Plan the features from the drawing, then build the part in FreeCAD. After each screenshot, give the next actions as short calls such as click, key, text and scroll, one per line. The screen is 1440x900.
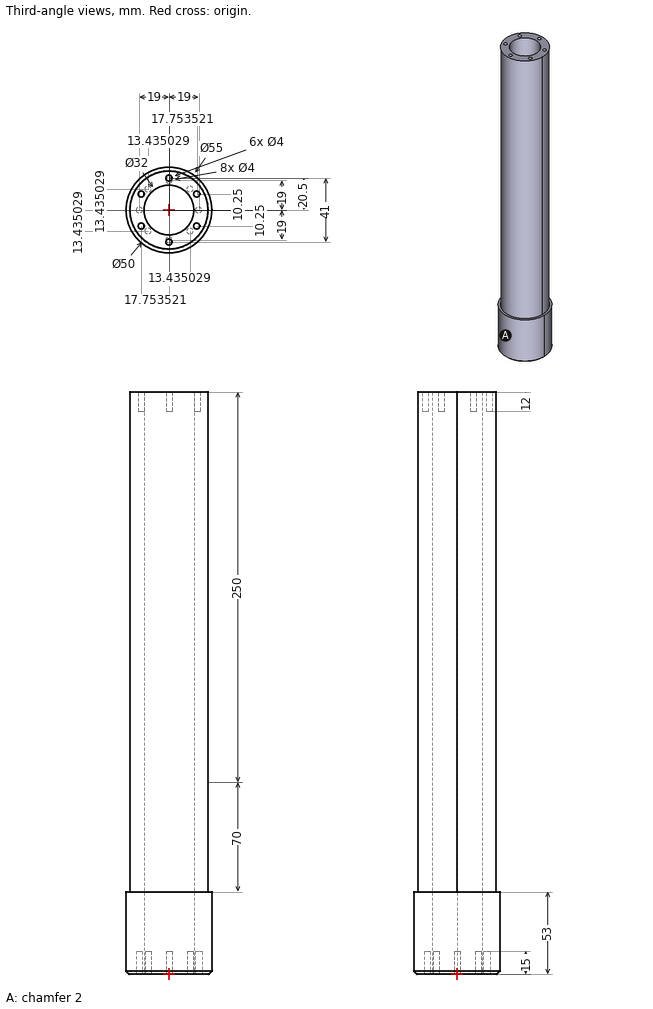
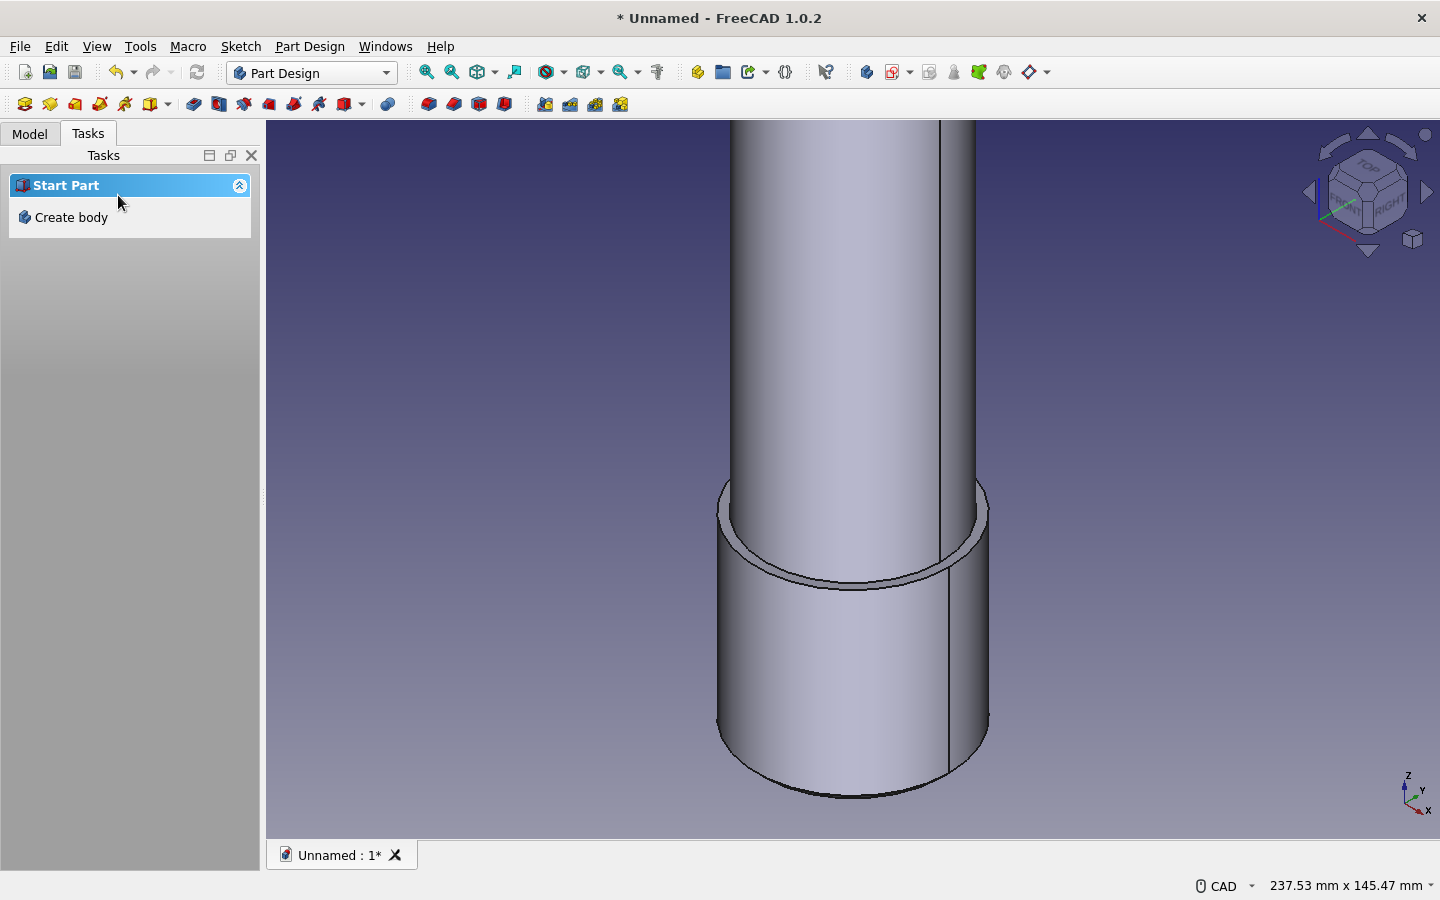
click(427, 72)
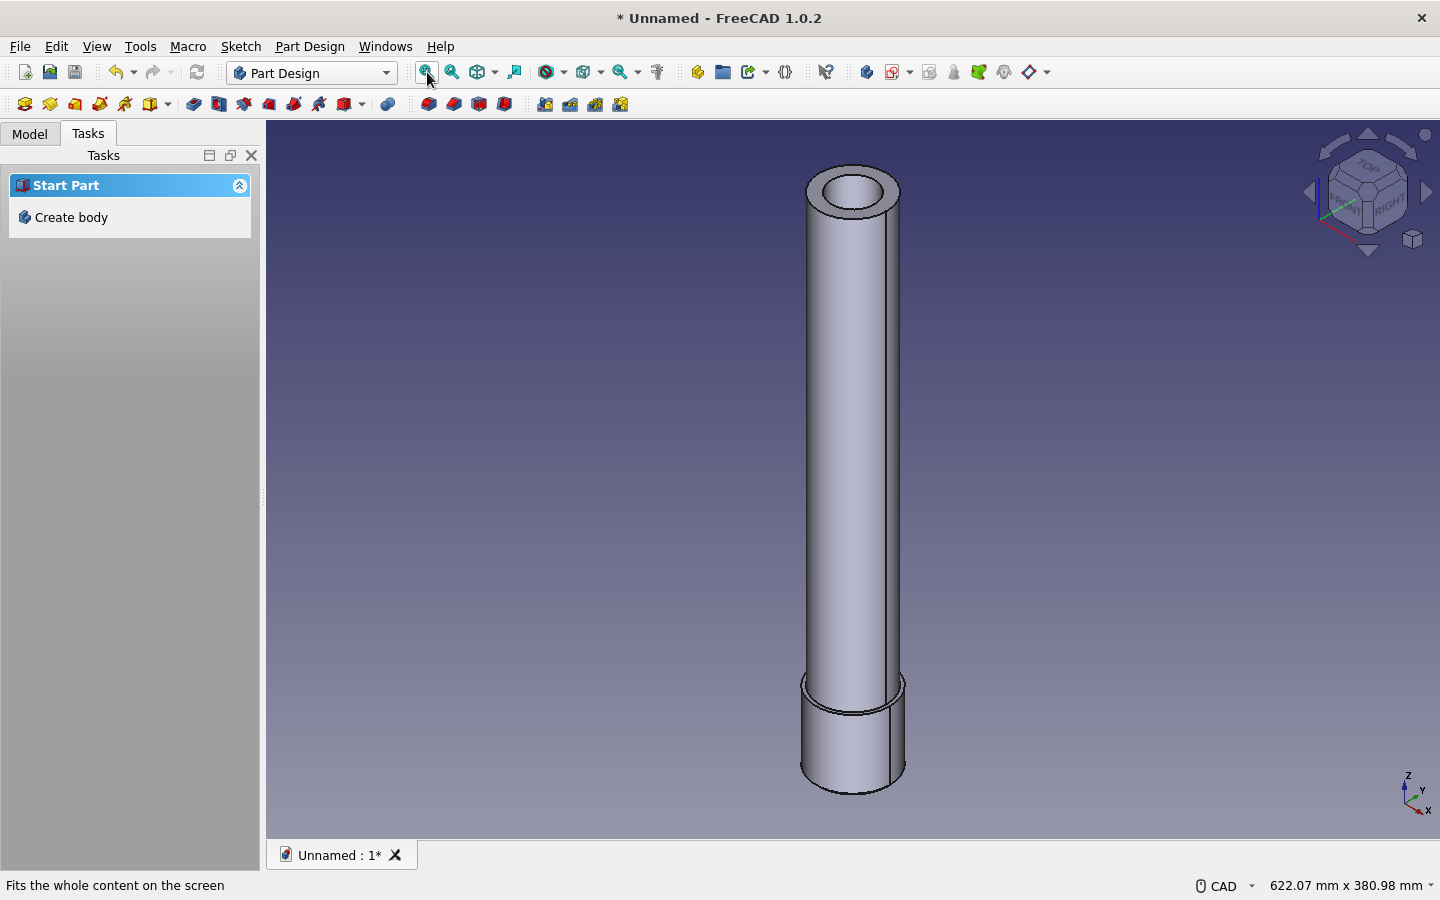
click(815, 191)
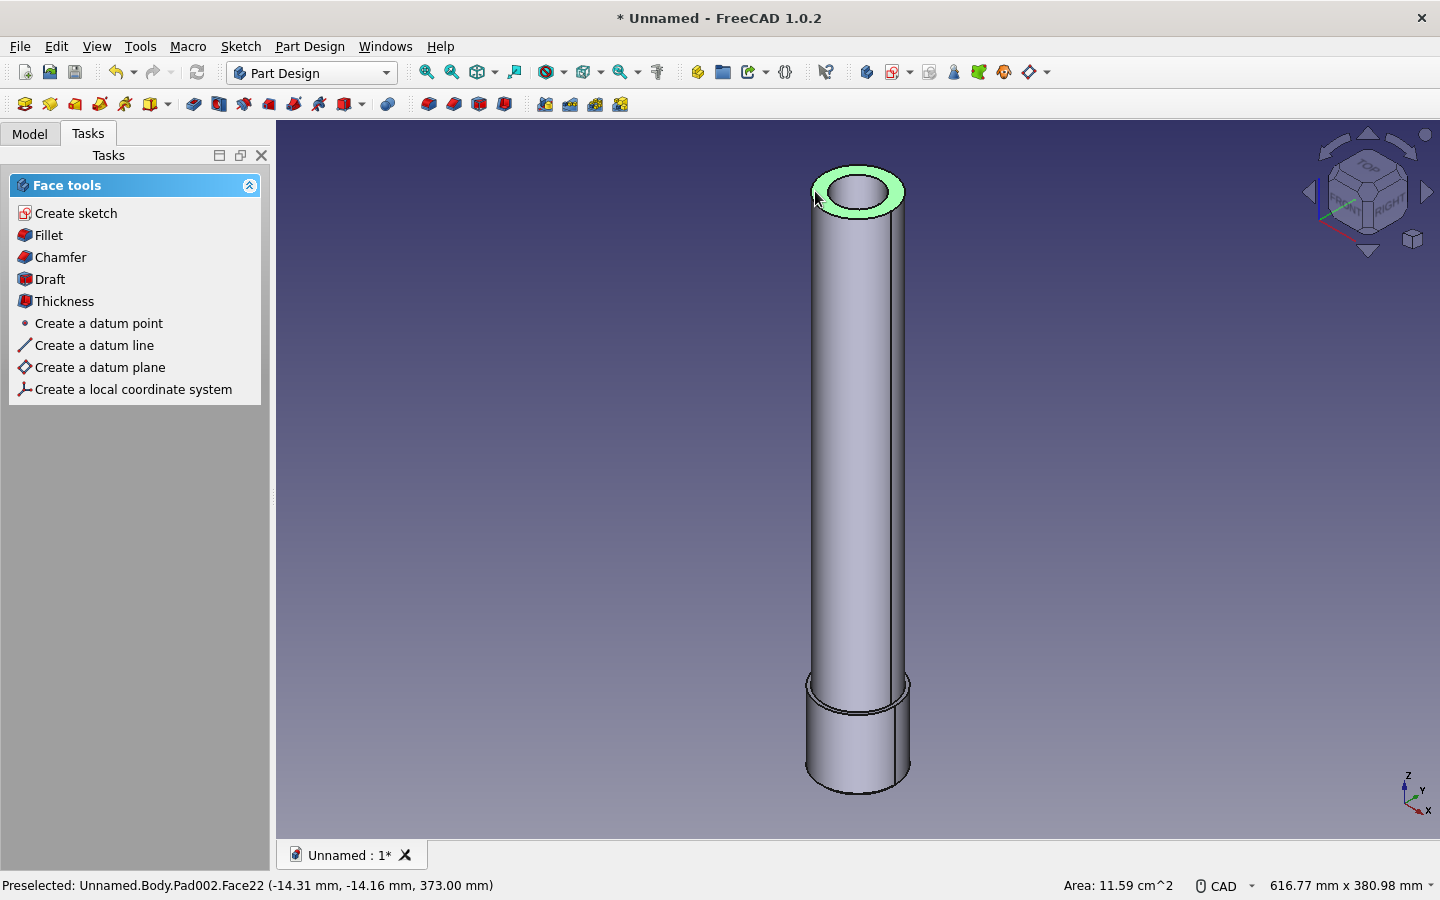
click(892, 72)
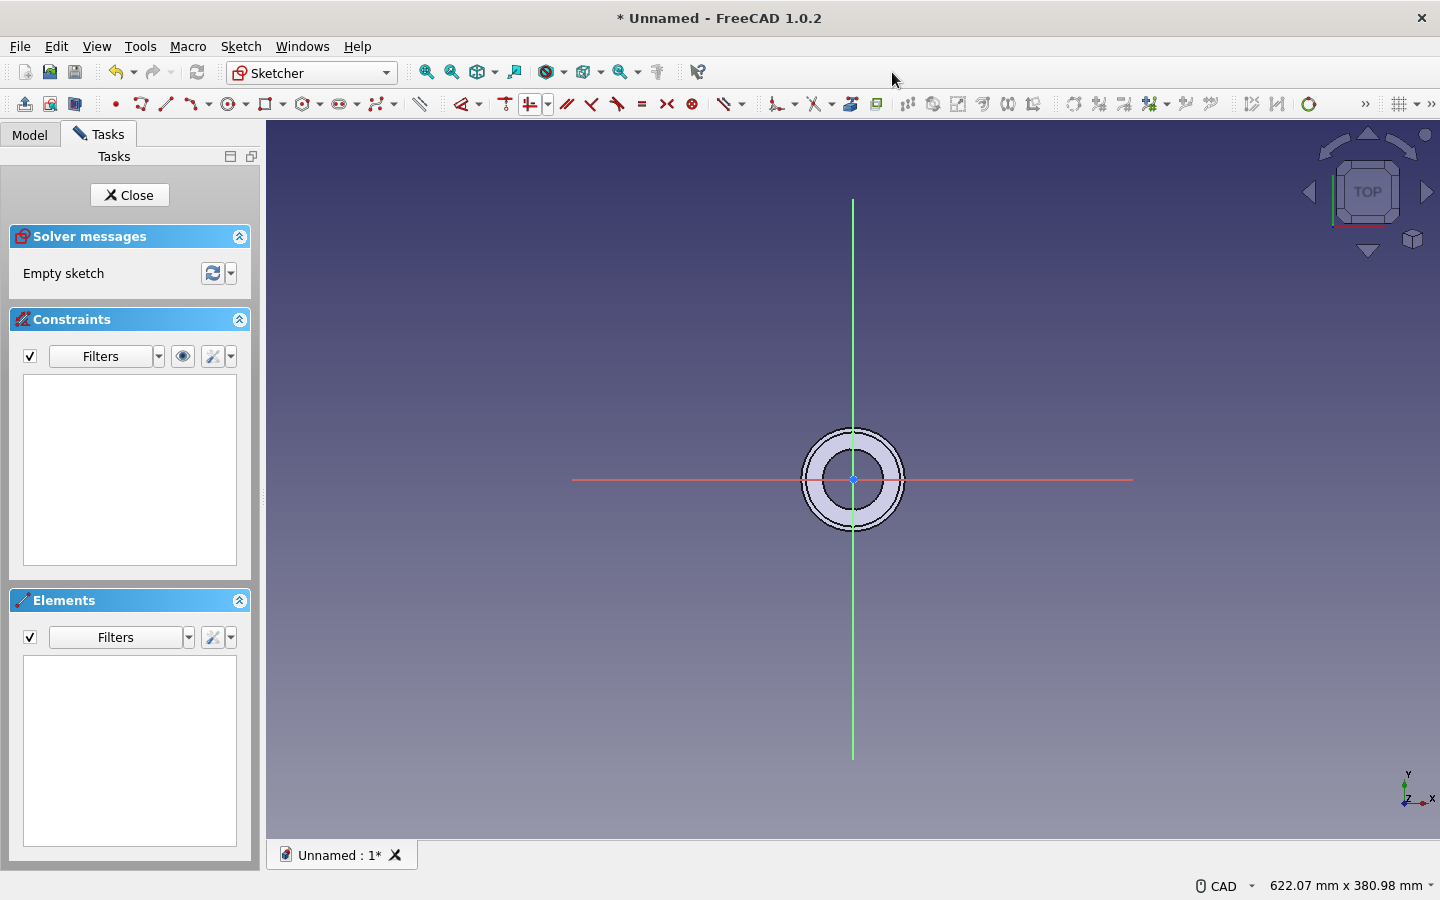
scroll(867, 480, up, 9)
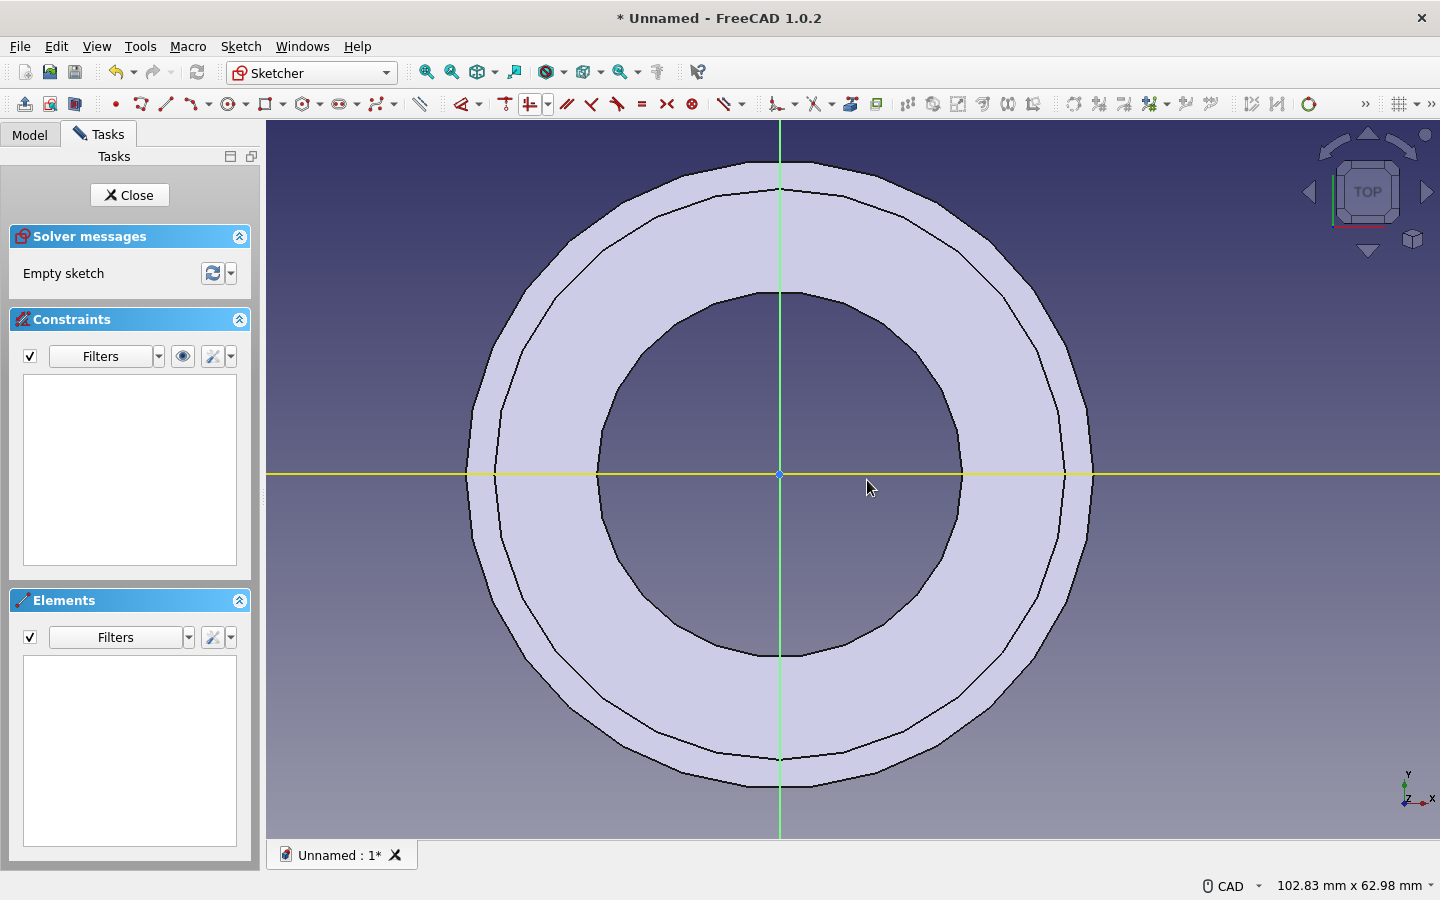
click(228, 104)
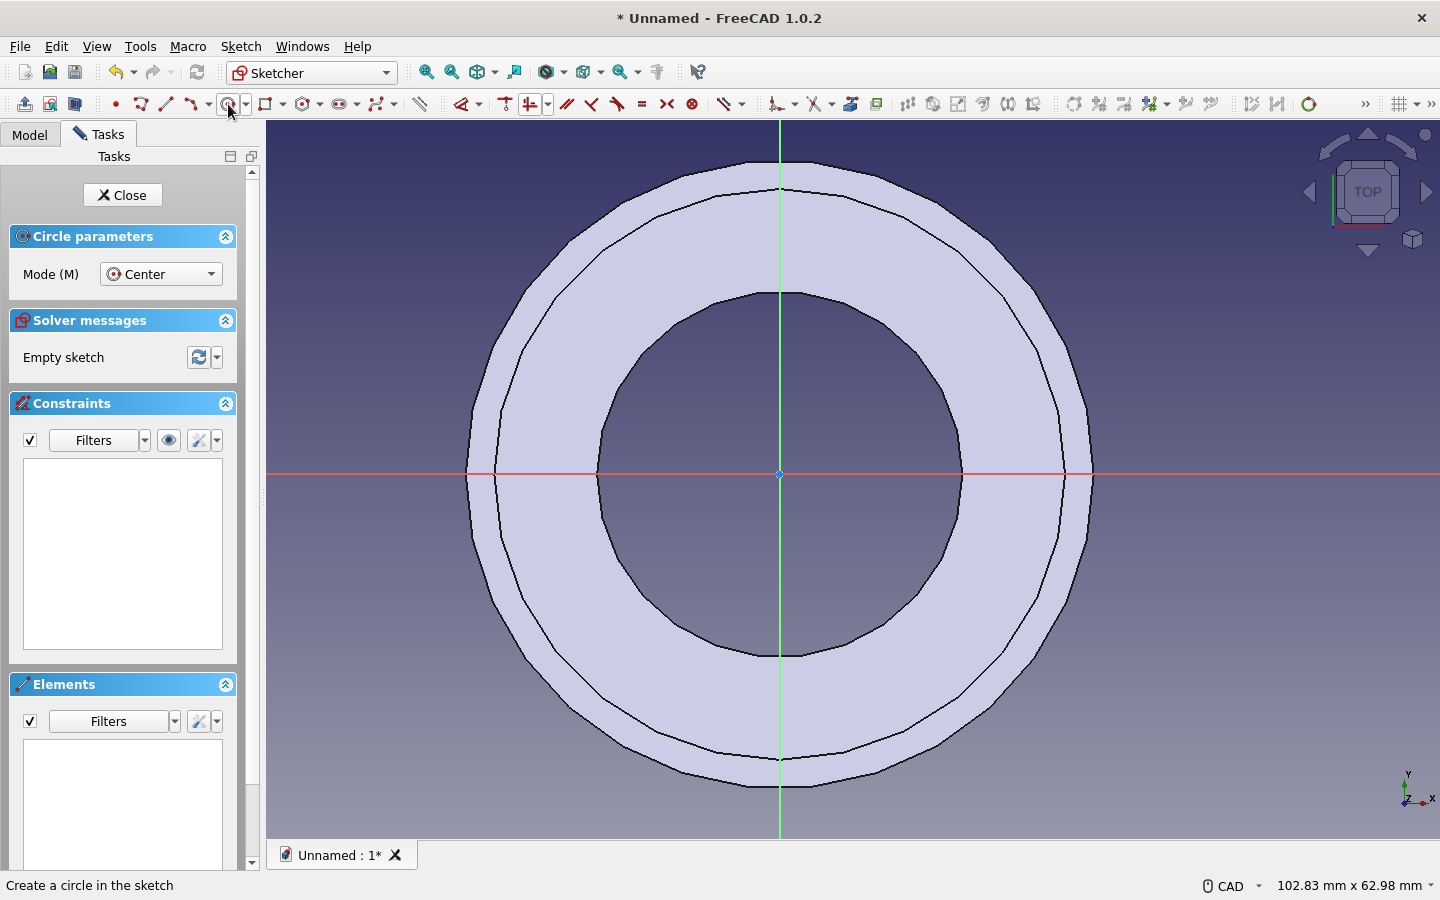
click(780, 240)
move(796, 224)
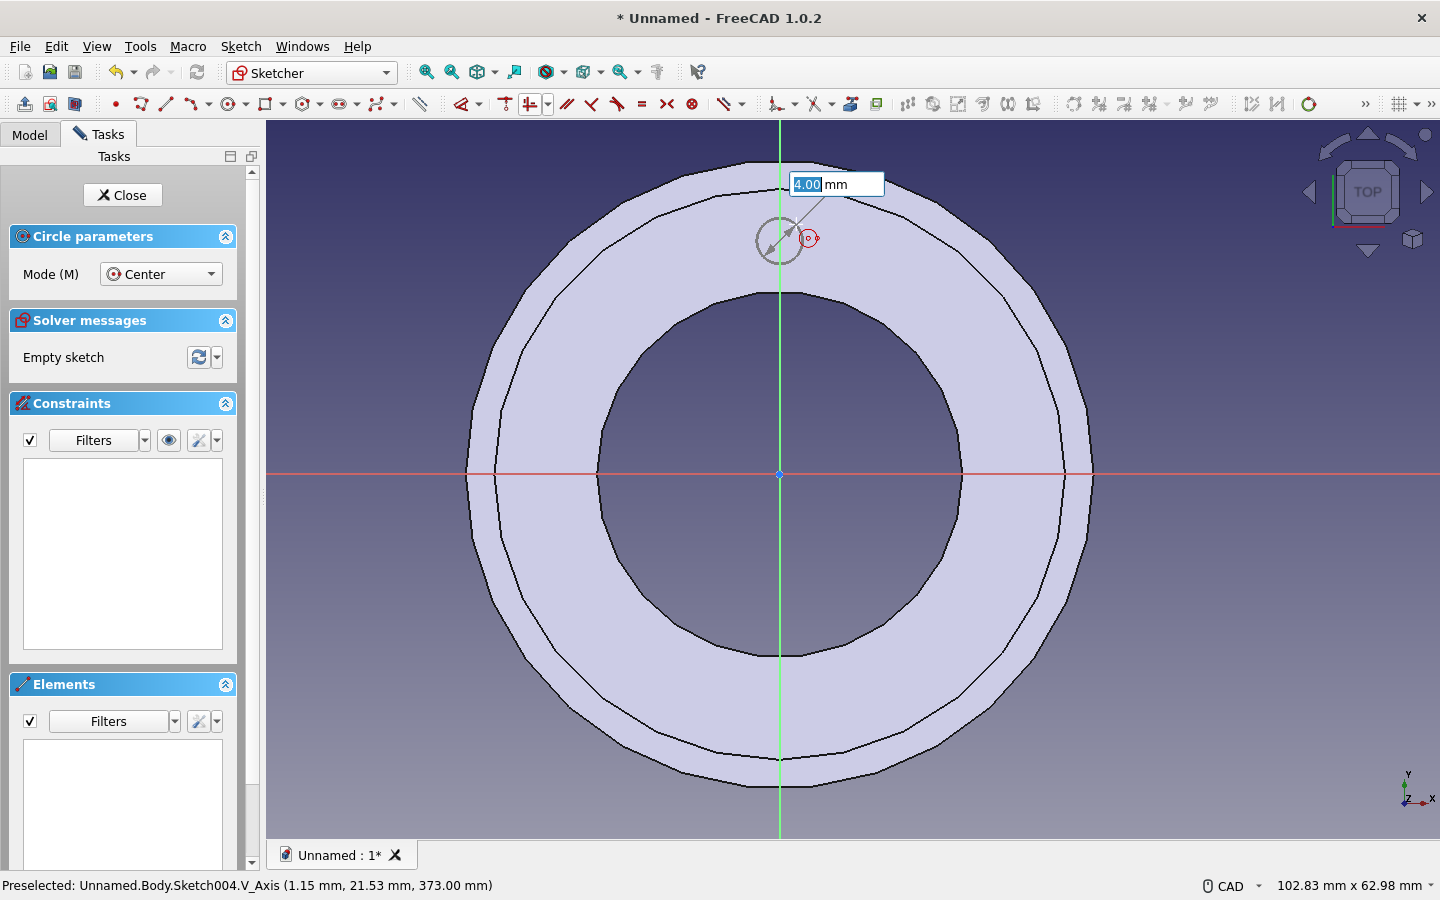
text(4)
key(Return)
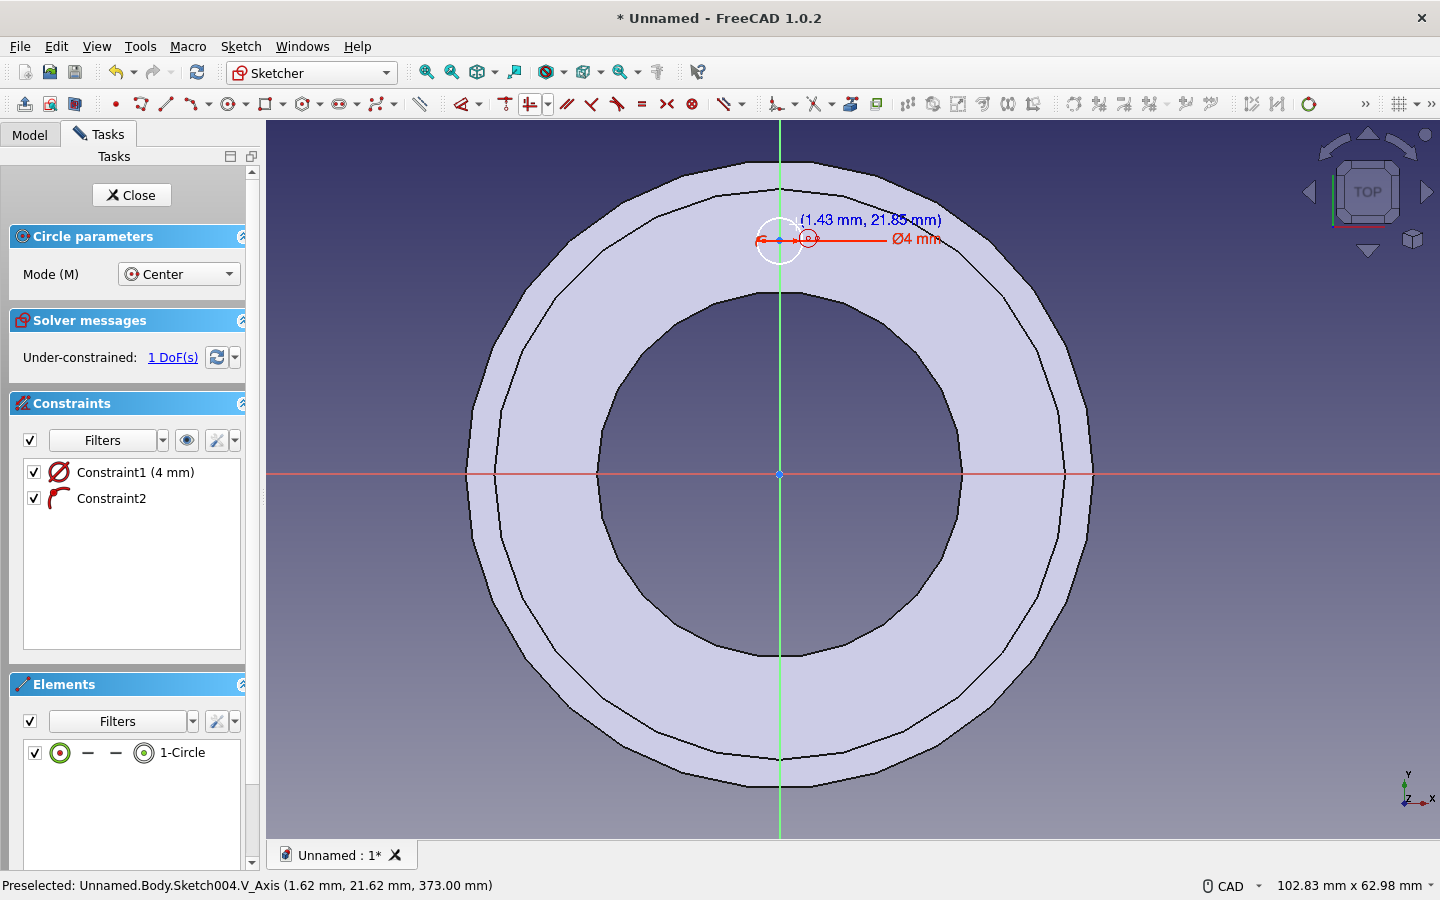
click(982, 357)
move(999, 341)